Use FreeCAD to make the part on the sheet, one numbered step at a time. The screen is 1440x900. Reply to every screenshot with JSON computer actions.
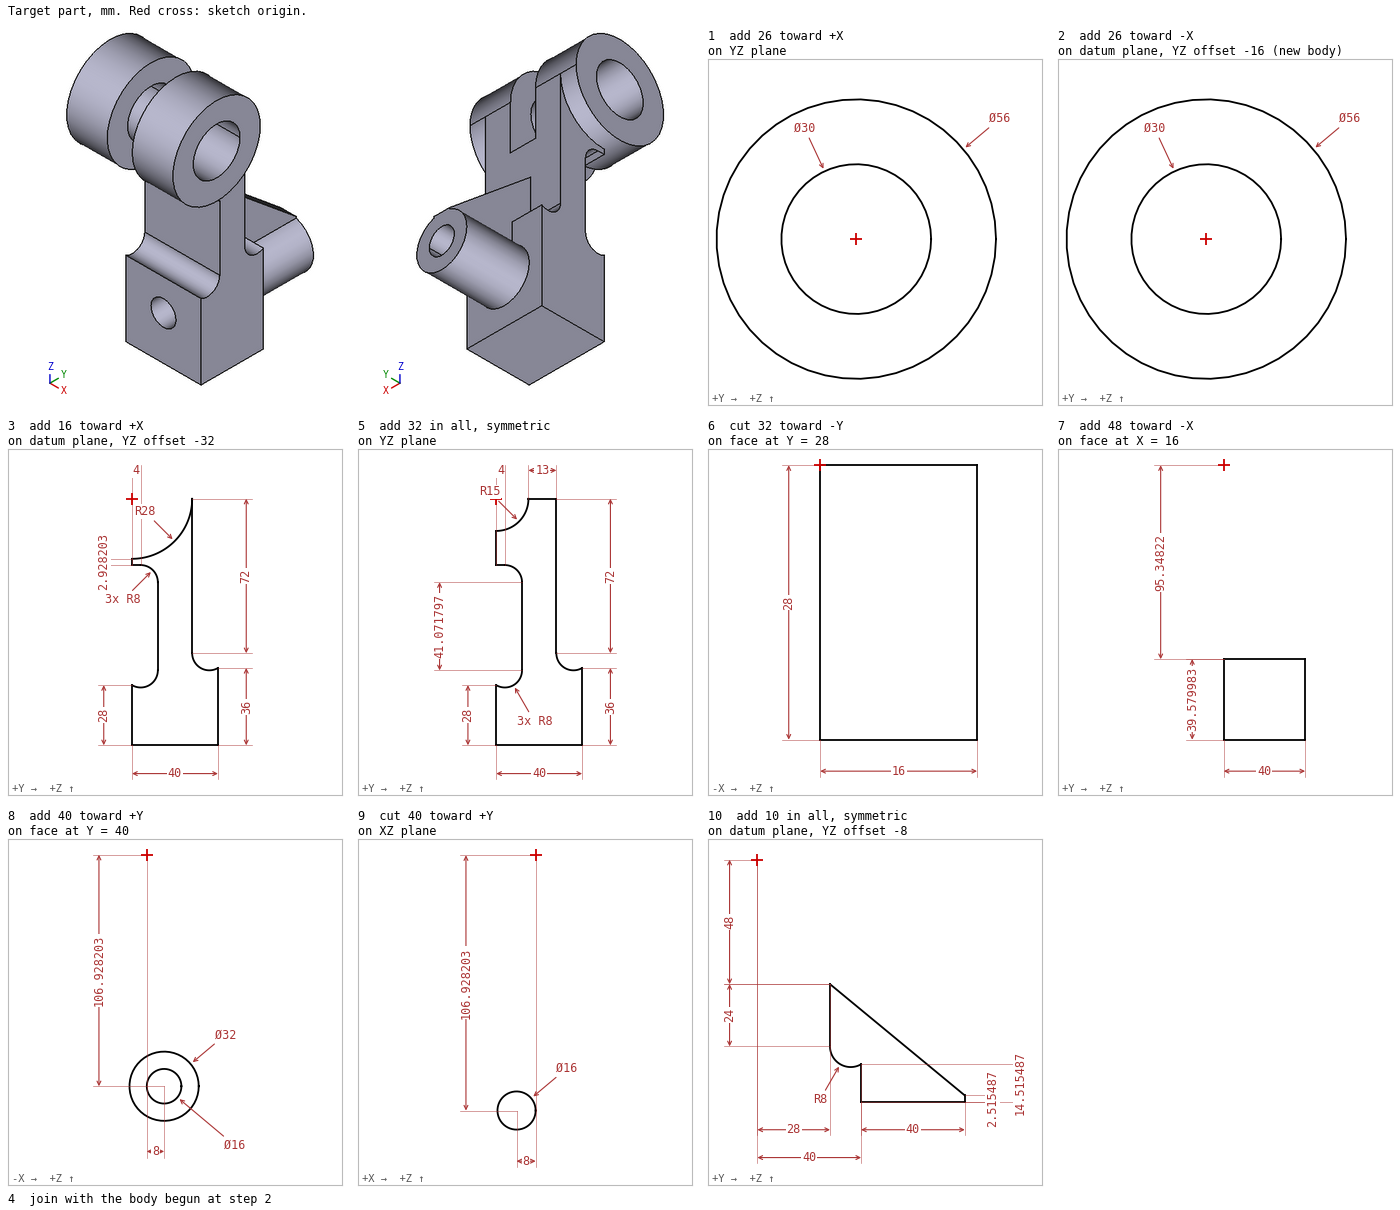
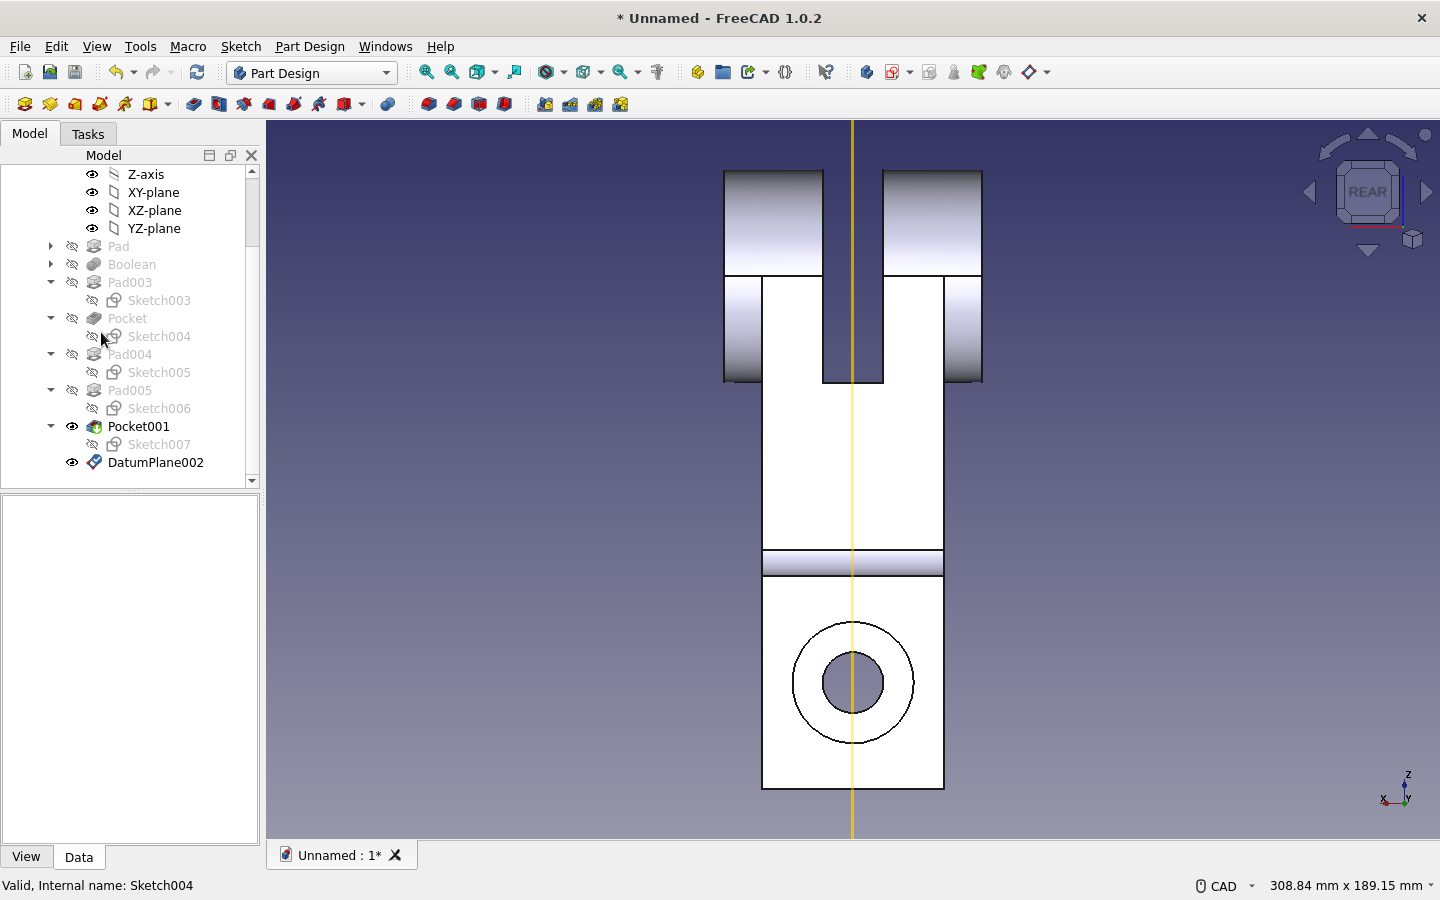
{"action": "left_click", "coordinate": [117, 462]}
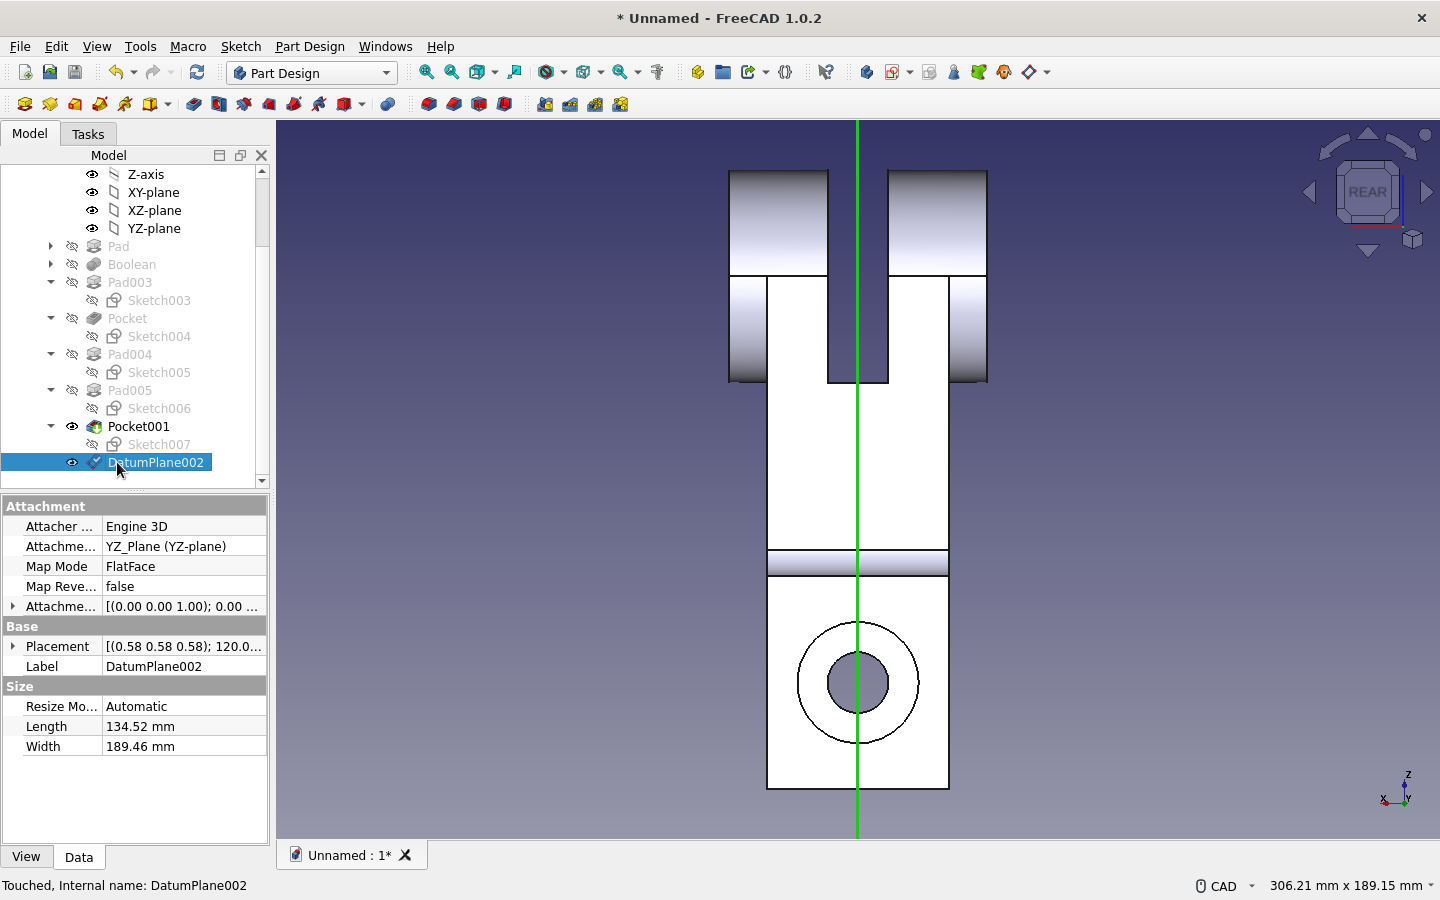
{"action": "left_click", "coordinate": [892, 72]}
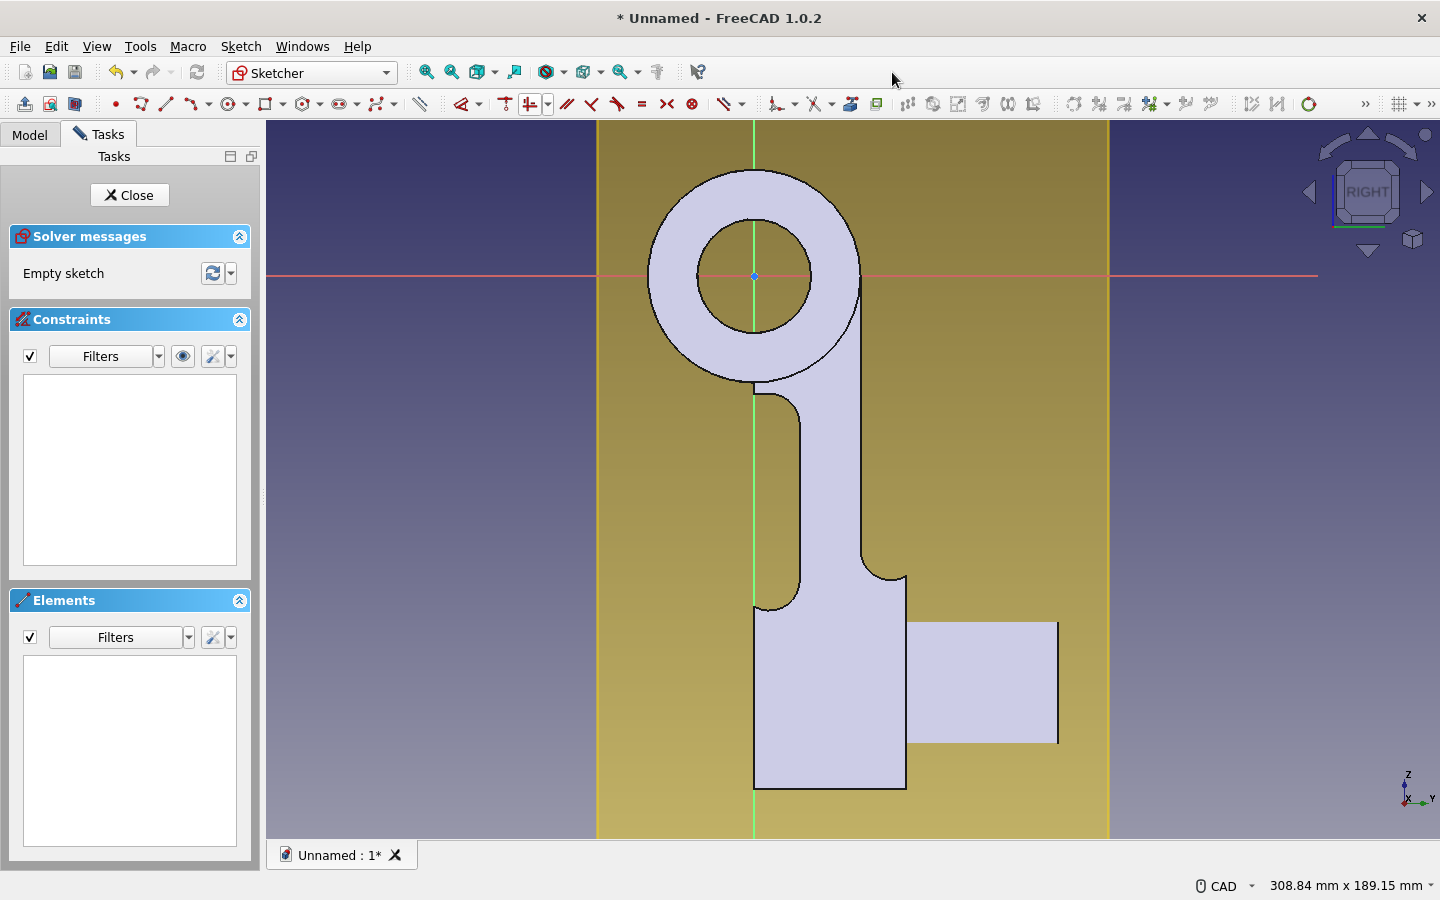
{"action": "key", "text": "q s"}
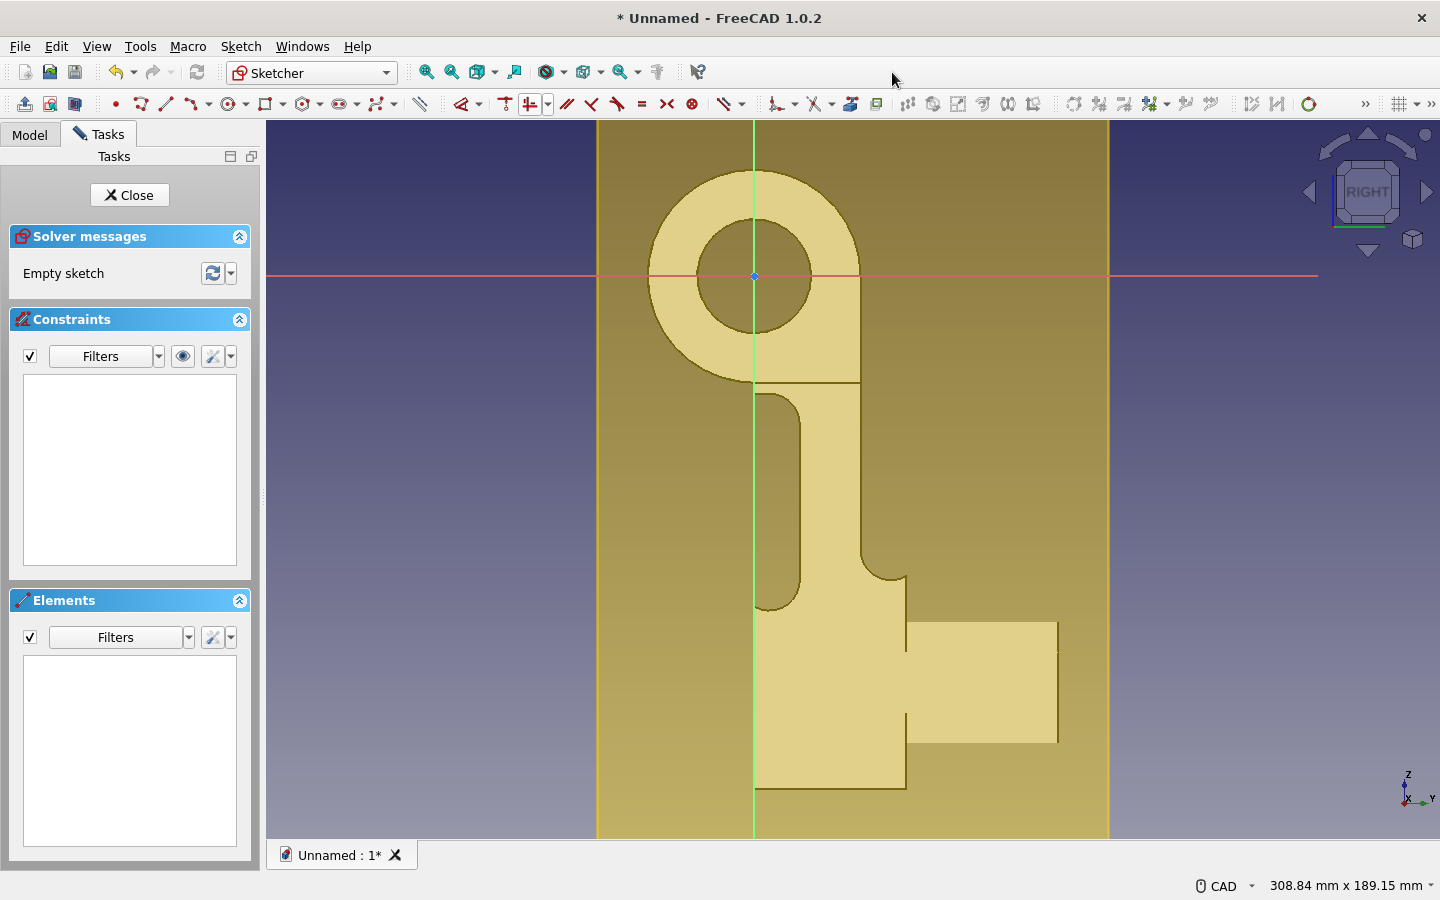
{"action": "left_click", "coordinate": [141, 104]}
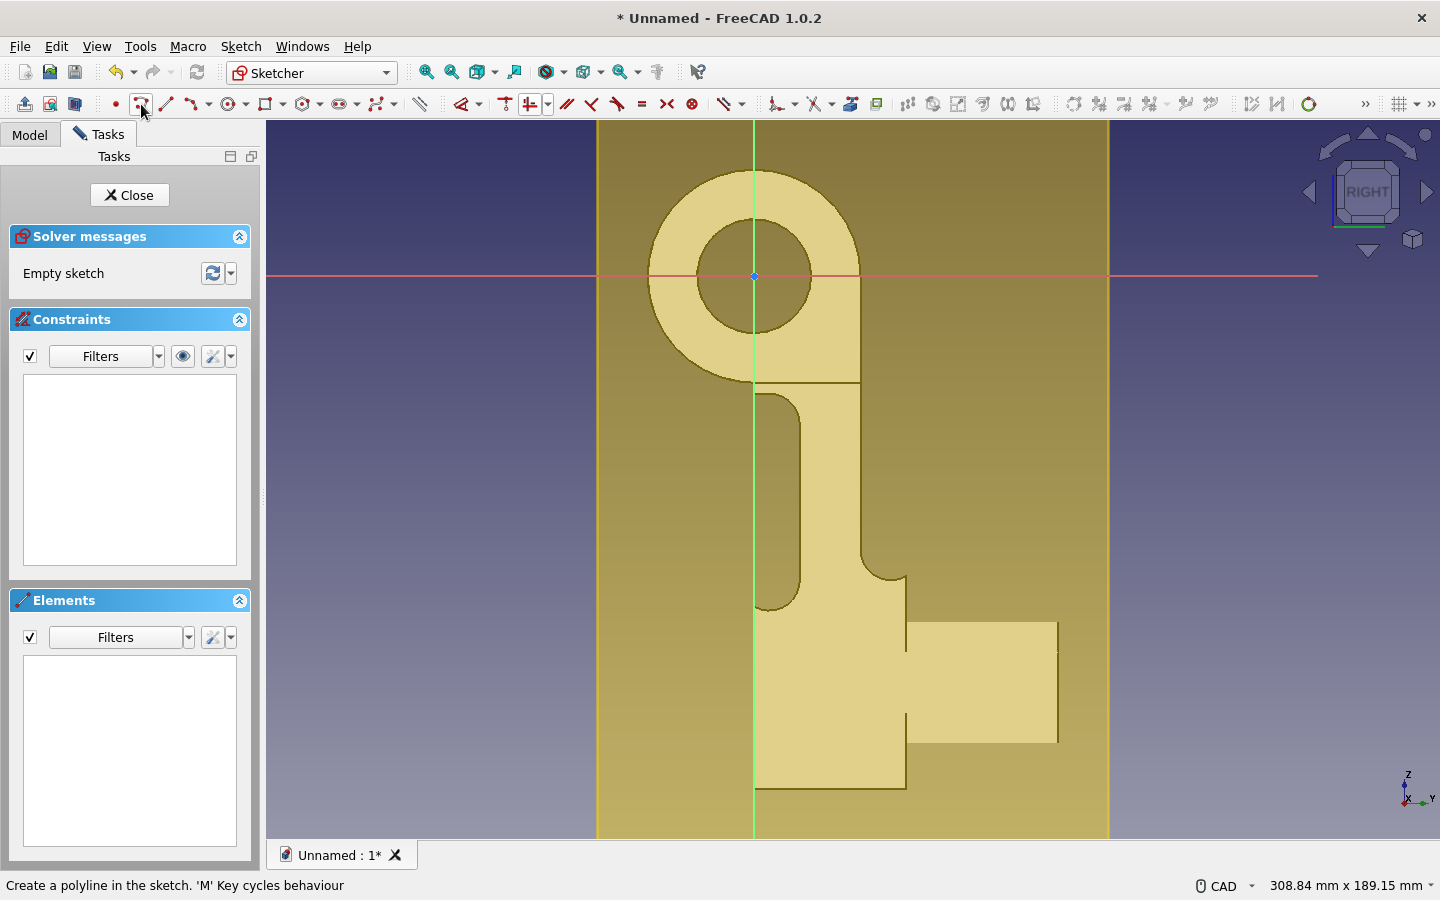
{"action": "left_click", "coordinate": [906, 576]}
{"action": "left_click", "coordinate": [906, 631]}
{"action": "left_click", "coordinate": [1058, 631]}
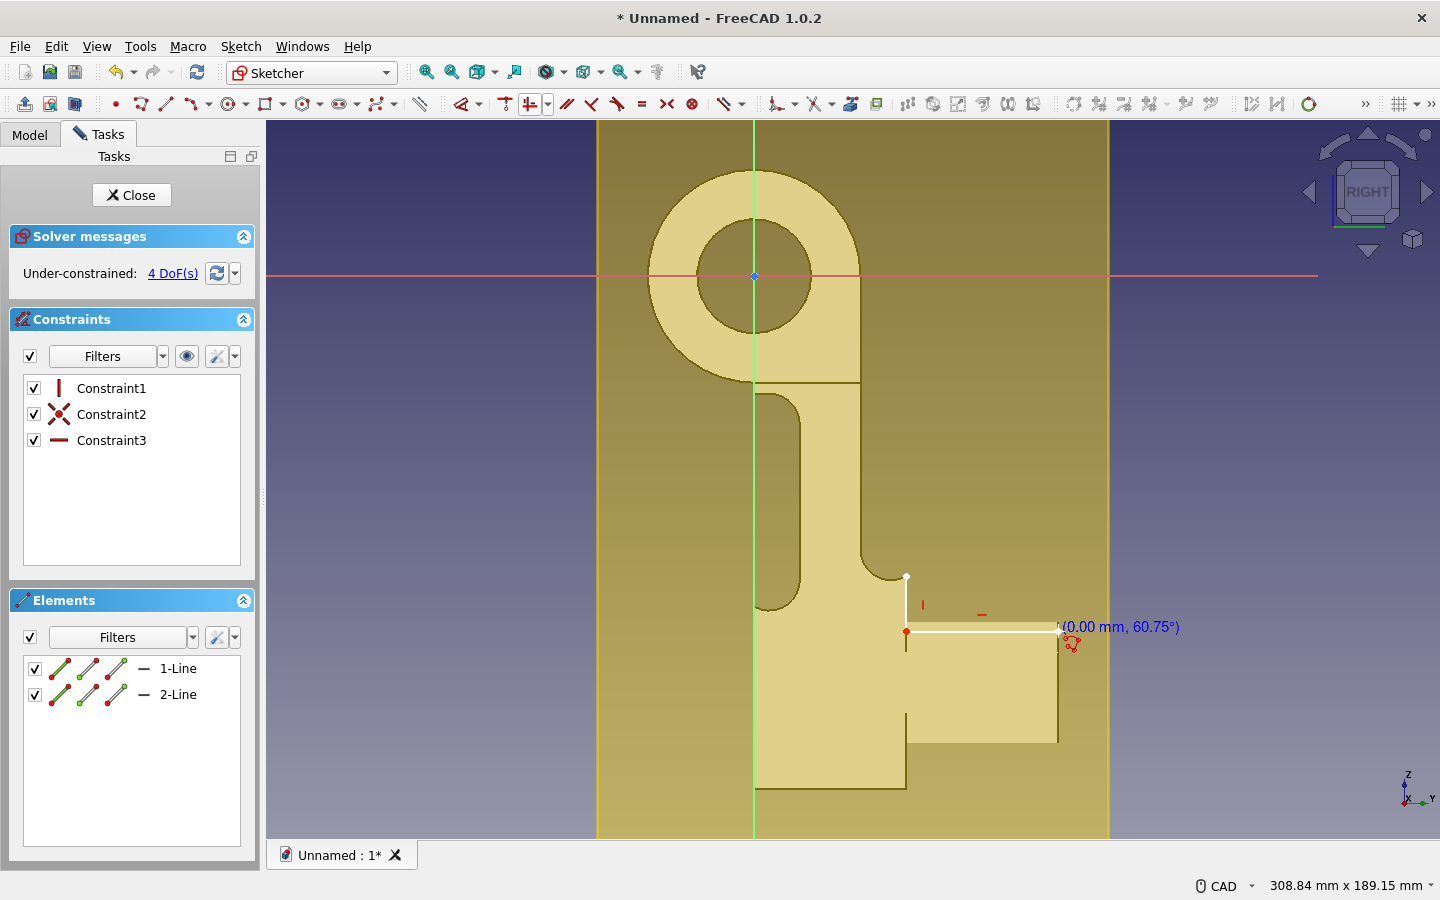
{"action": "scroll", "coordinate": [1058, 622], "scroll_direction": "up", "scroll_amount": 3}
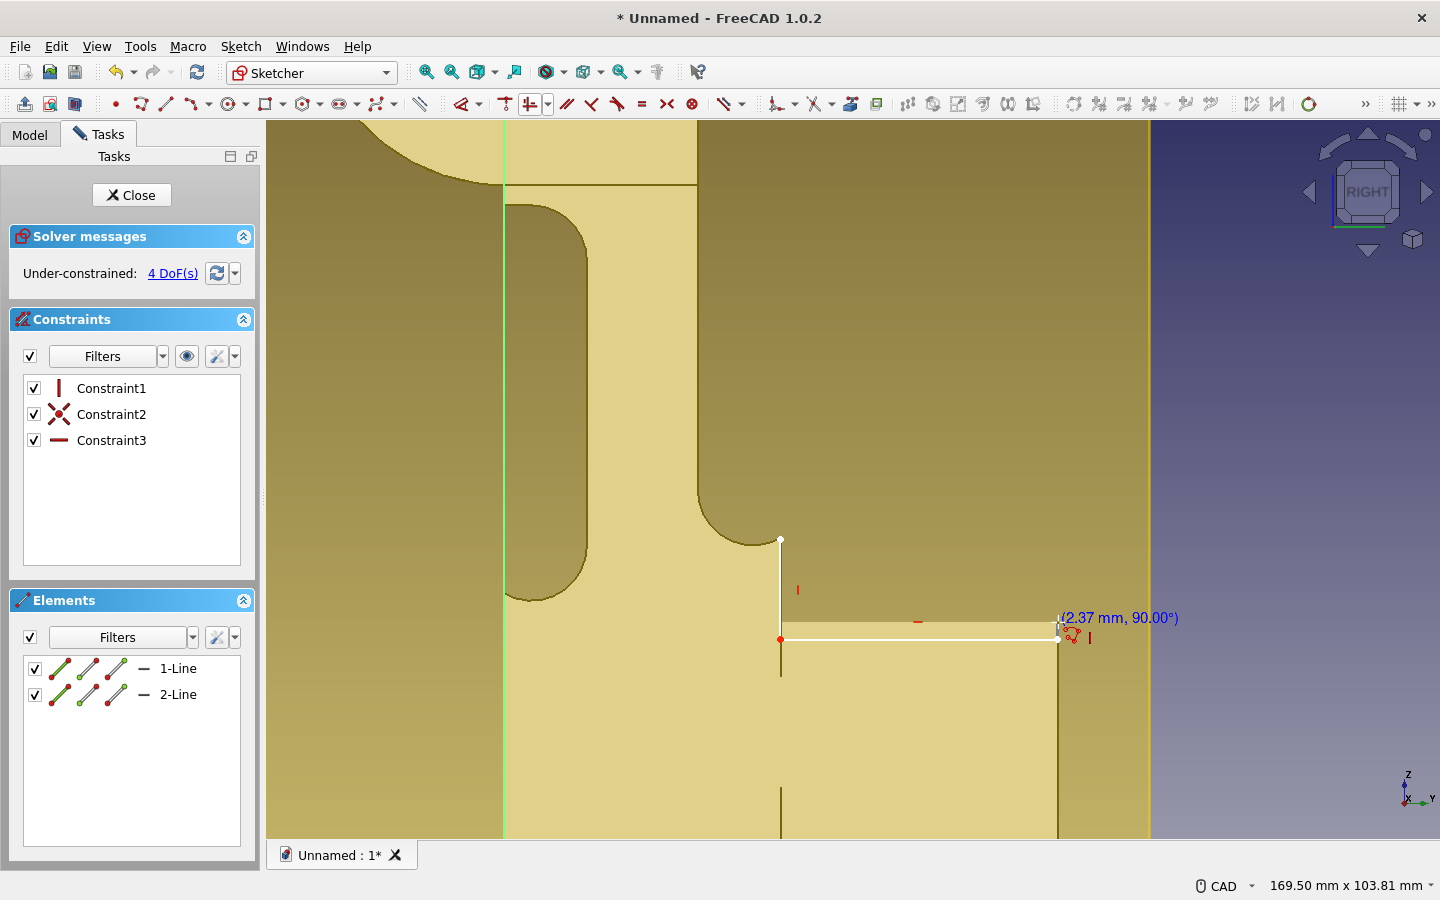
{"action": "left_click", "coordinate": [1057, 621]}
{"action": "left_click", "coordinate": [698, 324]}
{"action": "left_click", "coordinate": [698, 490]}
{"action": "right_click", "coordinate": [698, 490]}